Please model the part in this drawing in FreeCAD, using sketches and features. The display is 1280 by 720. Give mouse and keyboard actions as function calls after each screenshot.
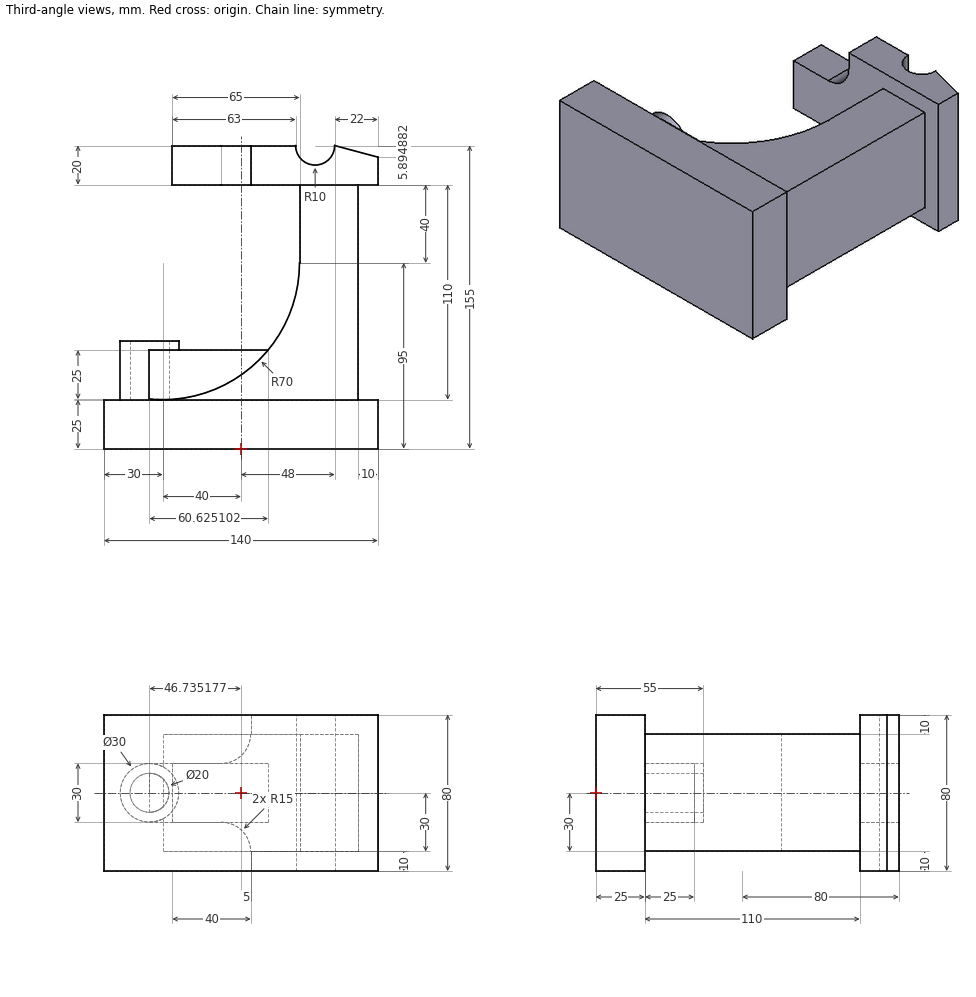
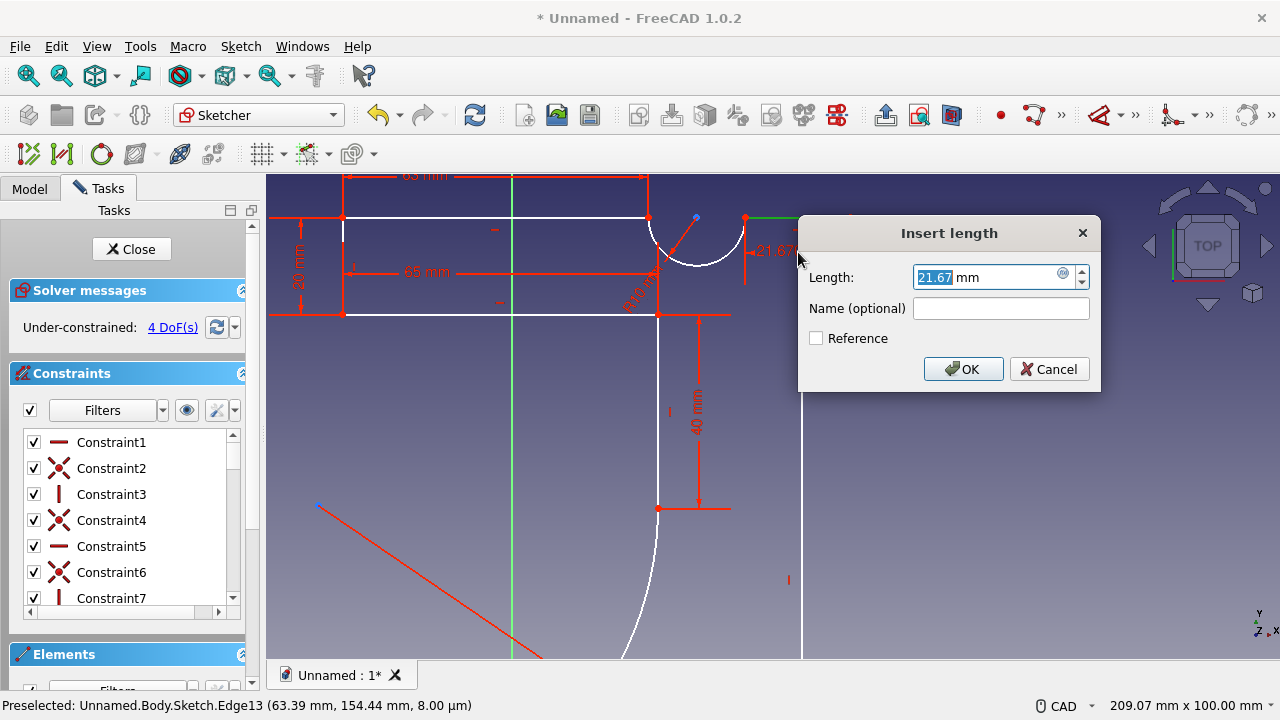
text(22)
key(Return)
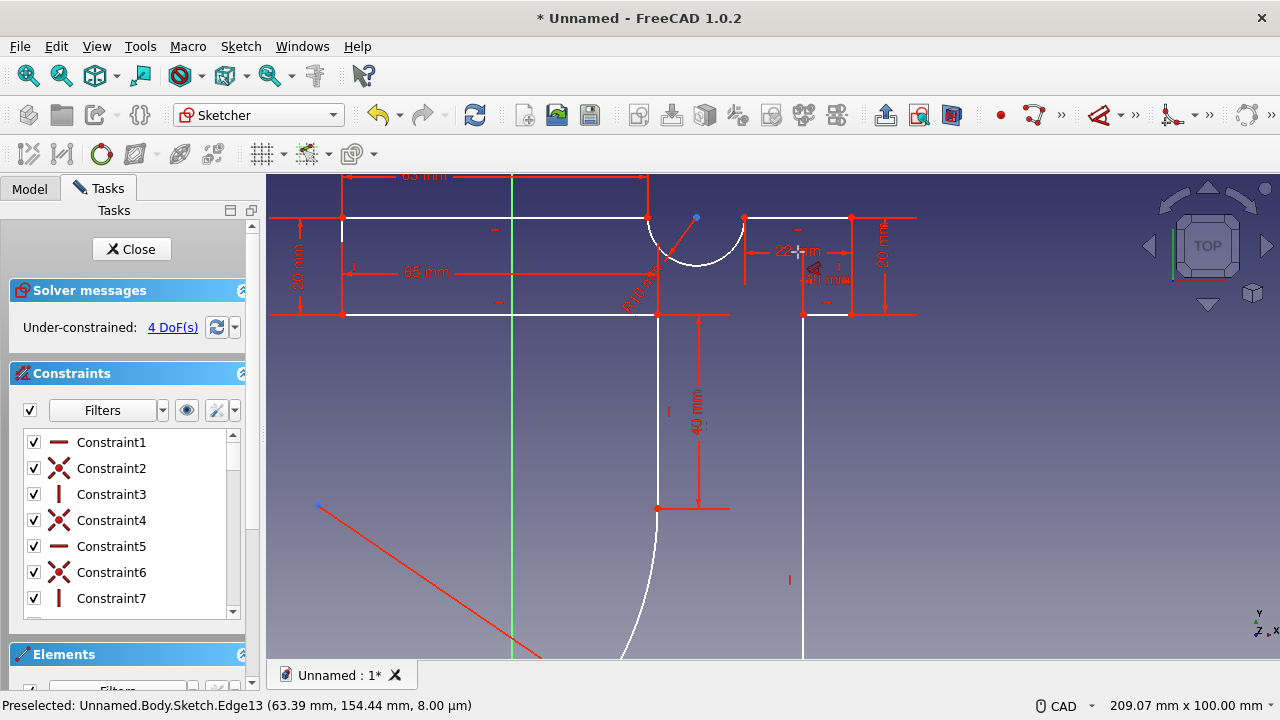
scroll(817, 315, down, 5)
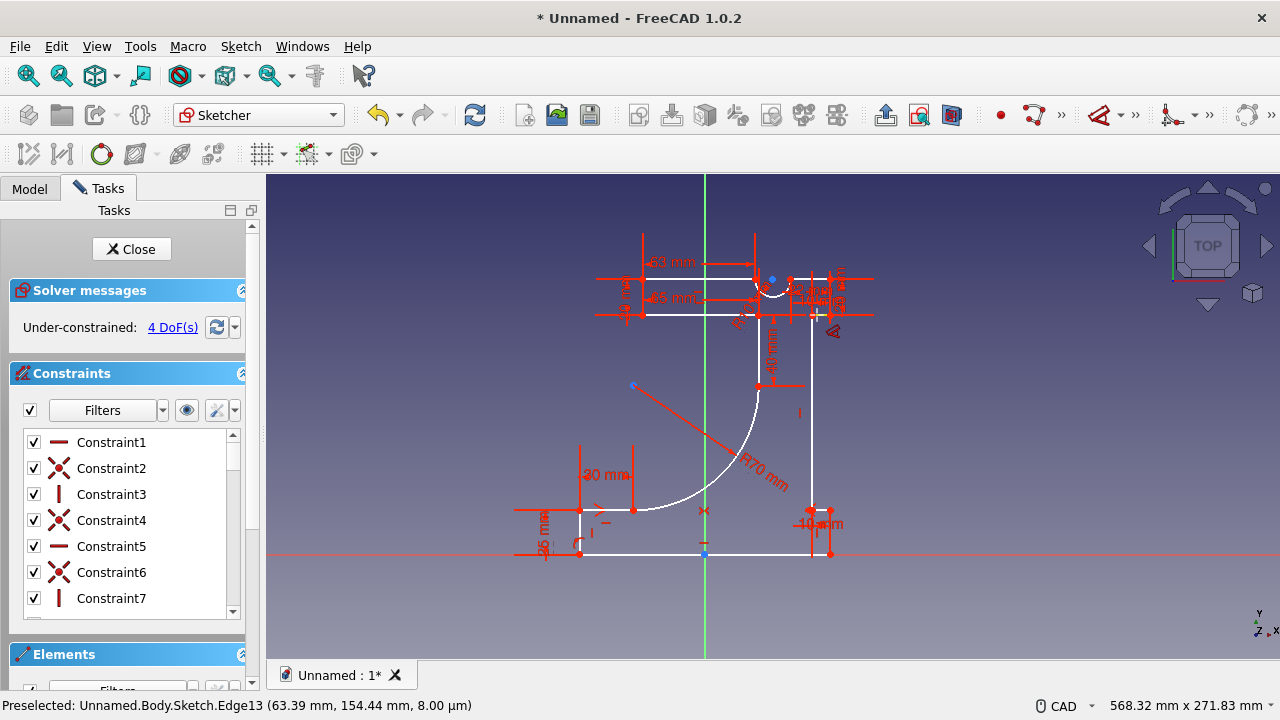
click(655, 555)
click(647, 589)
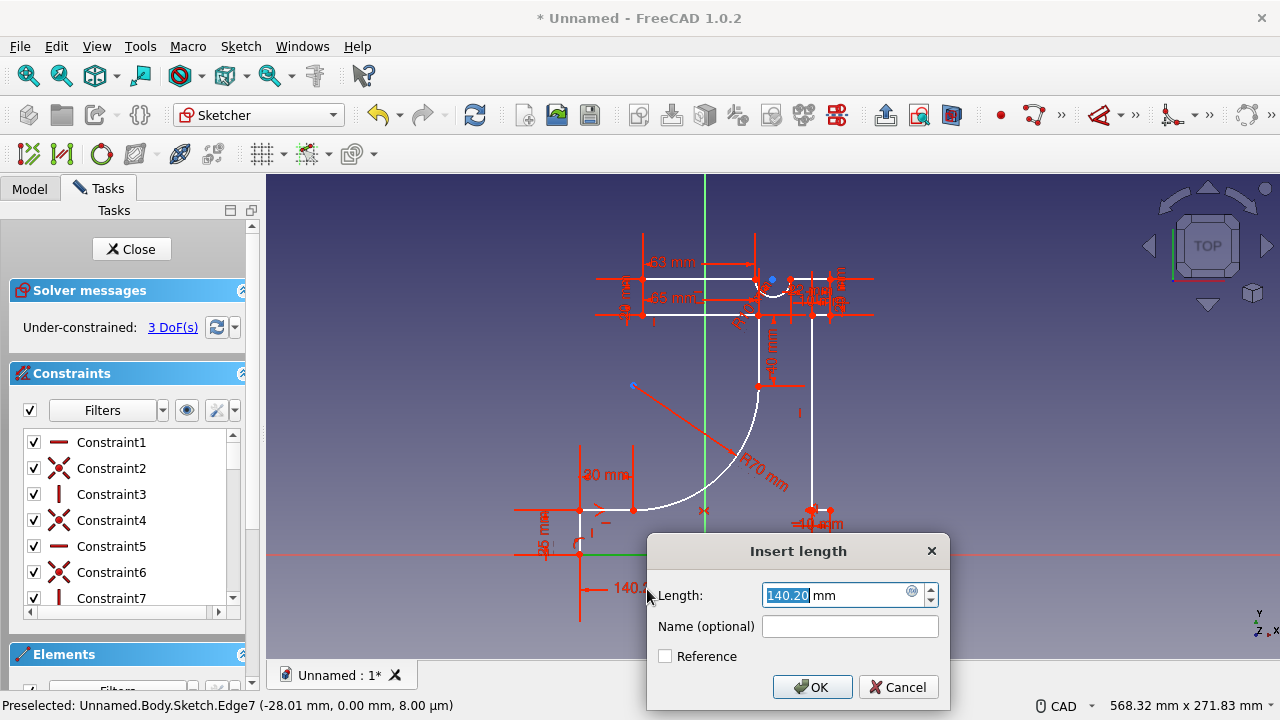
text(140)
key(Return)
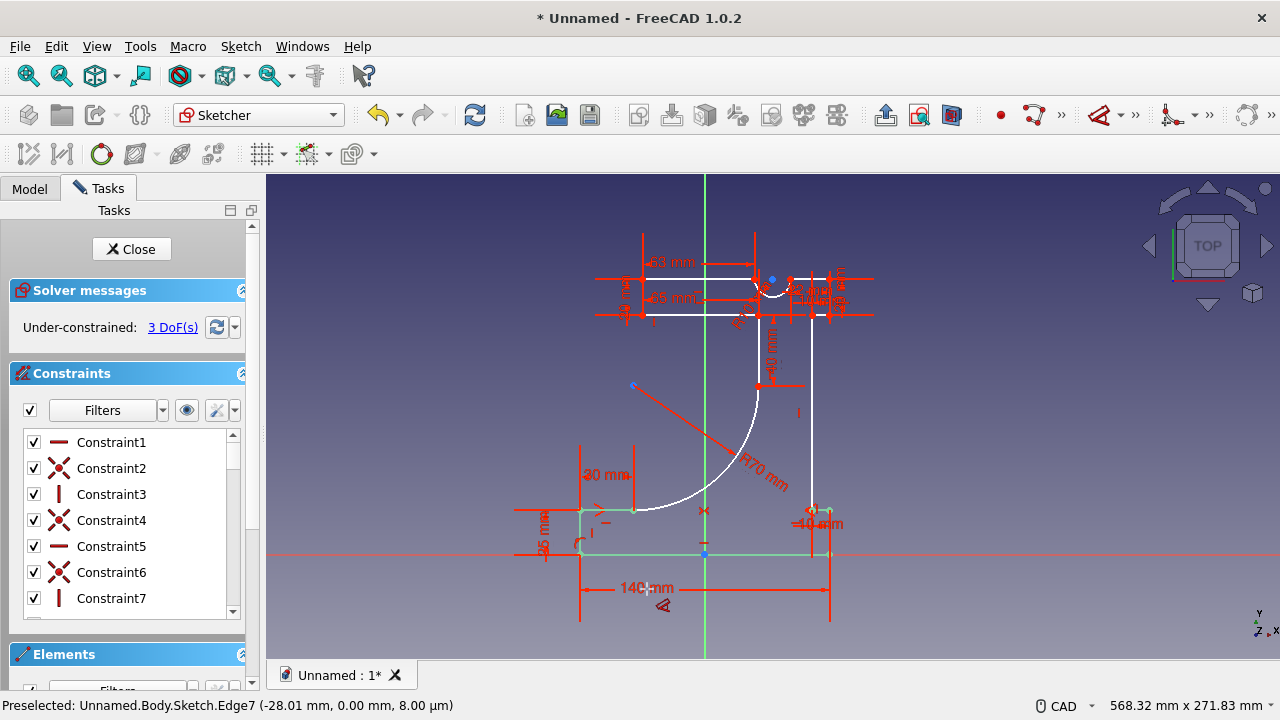
click(812, 452)
click(846, 413)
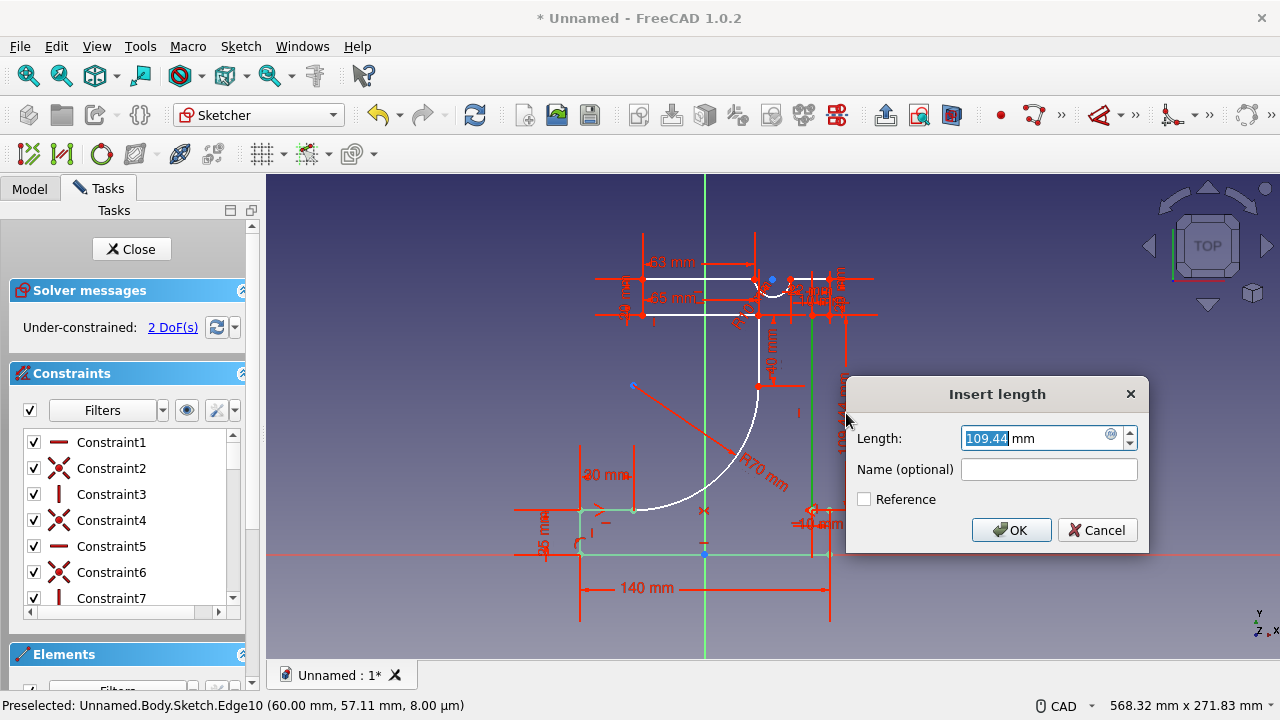
text(110)
key(Return)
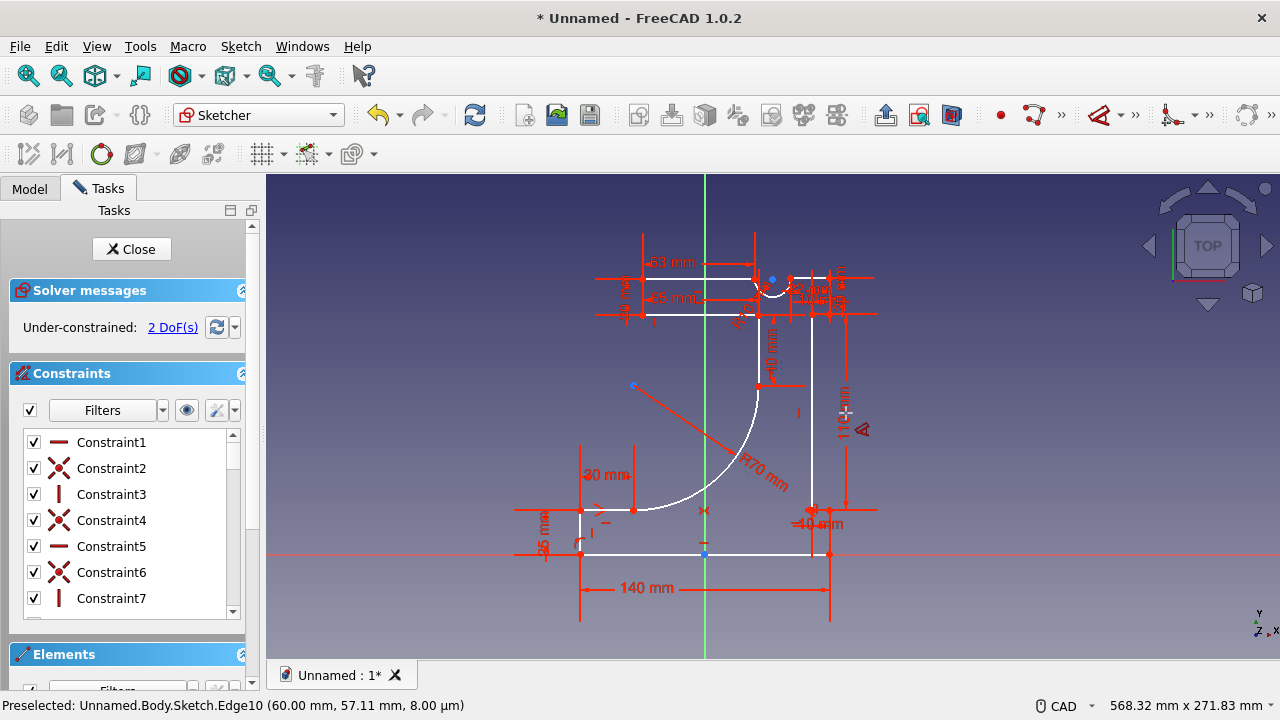
click(759, 386)
click(671, 432)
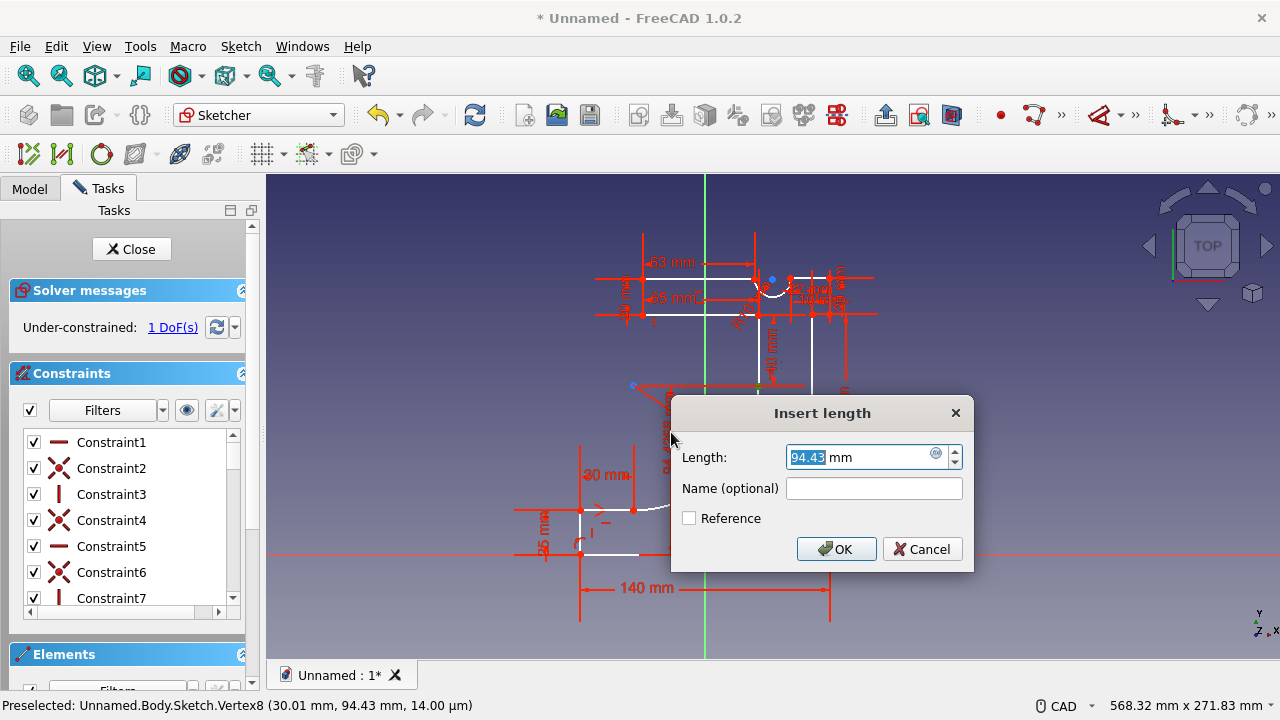
text(95)
key(Return)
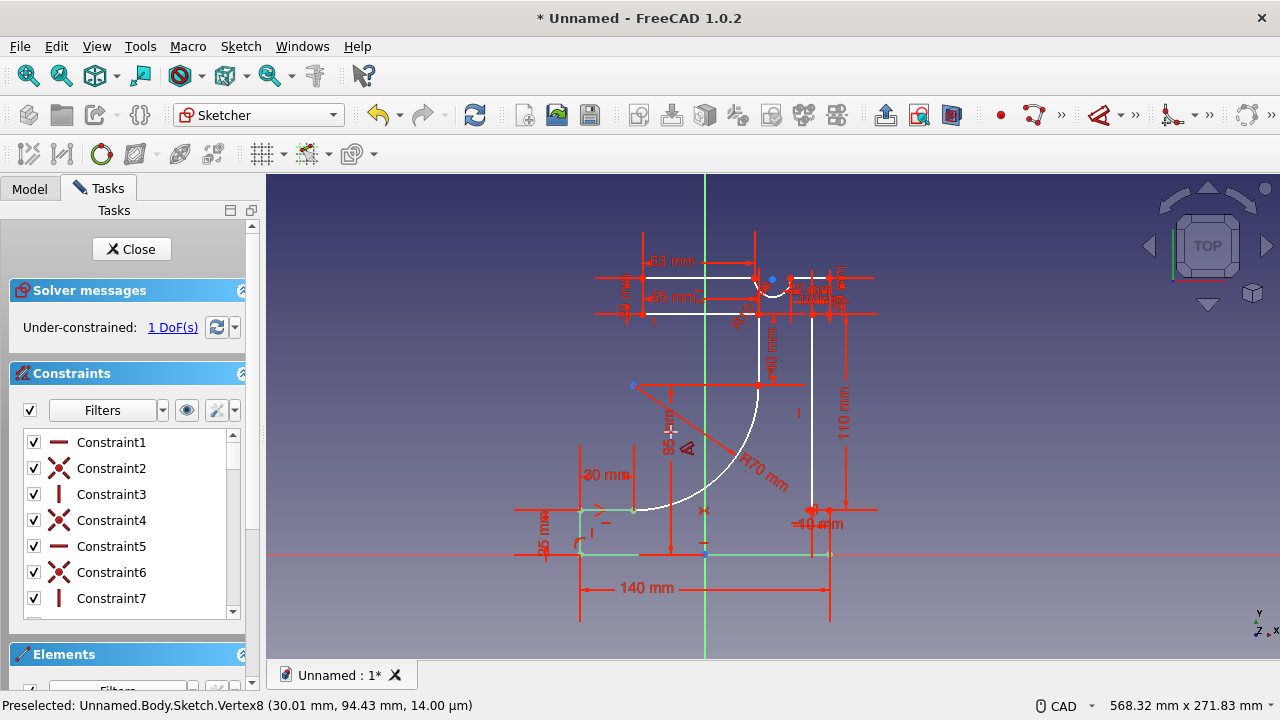
click(773, 279)
click(671, 354)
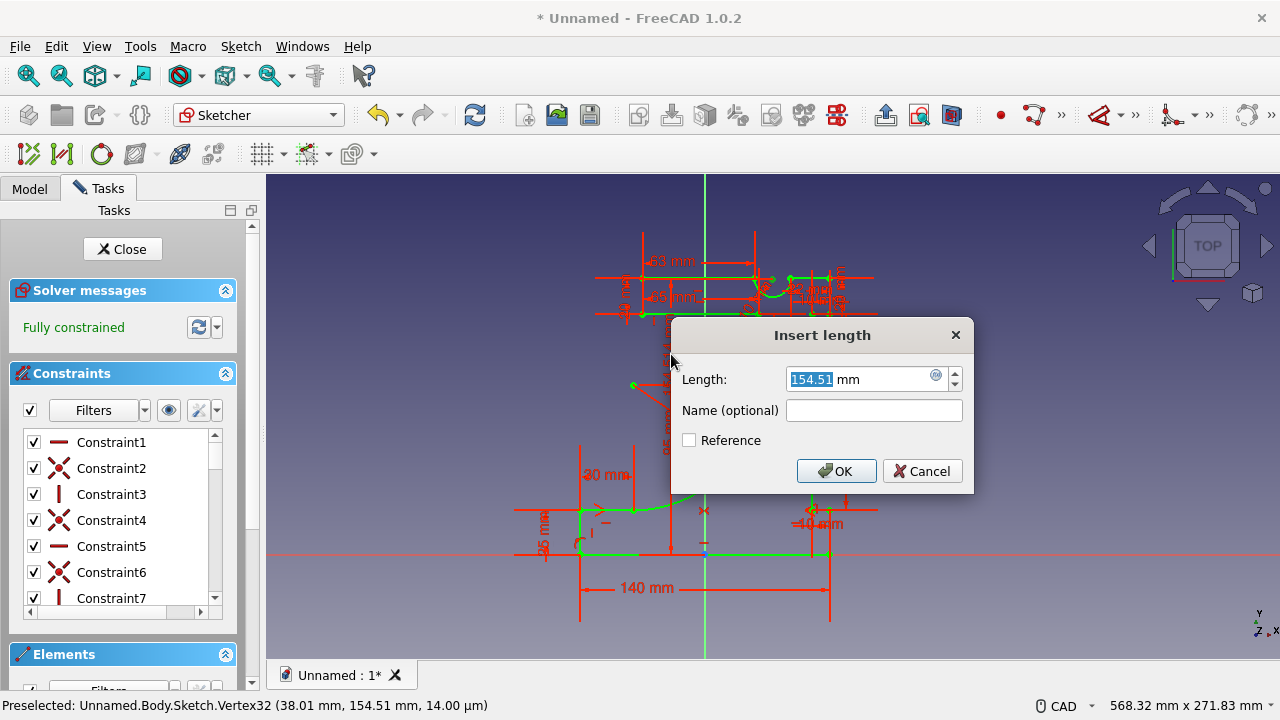
text(155)
key(Return)
key(Escape)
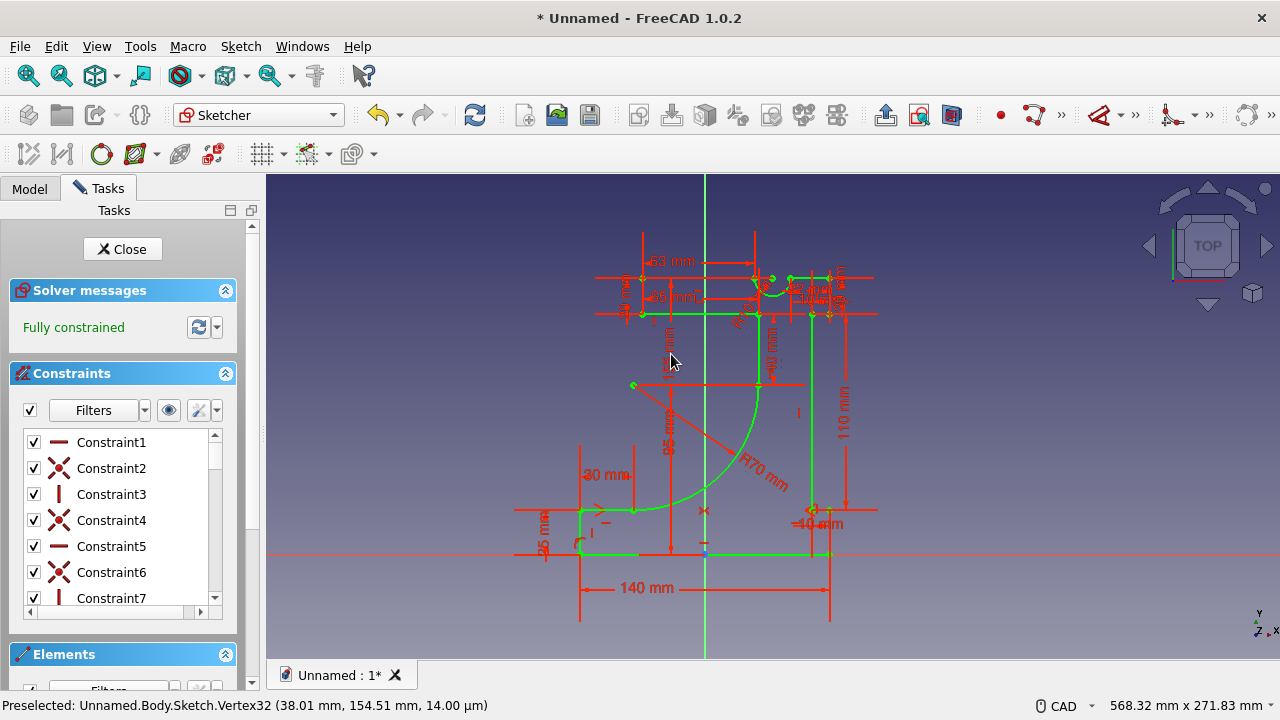
click(123, 249)